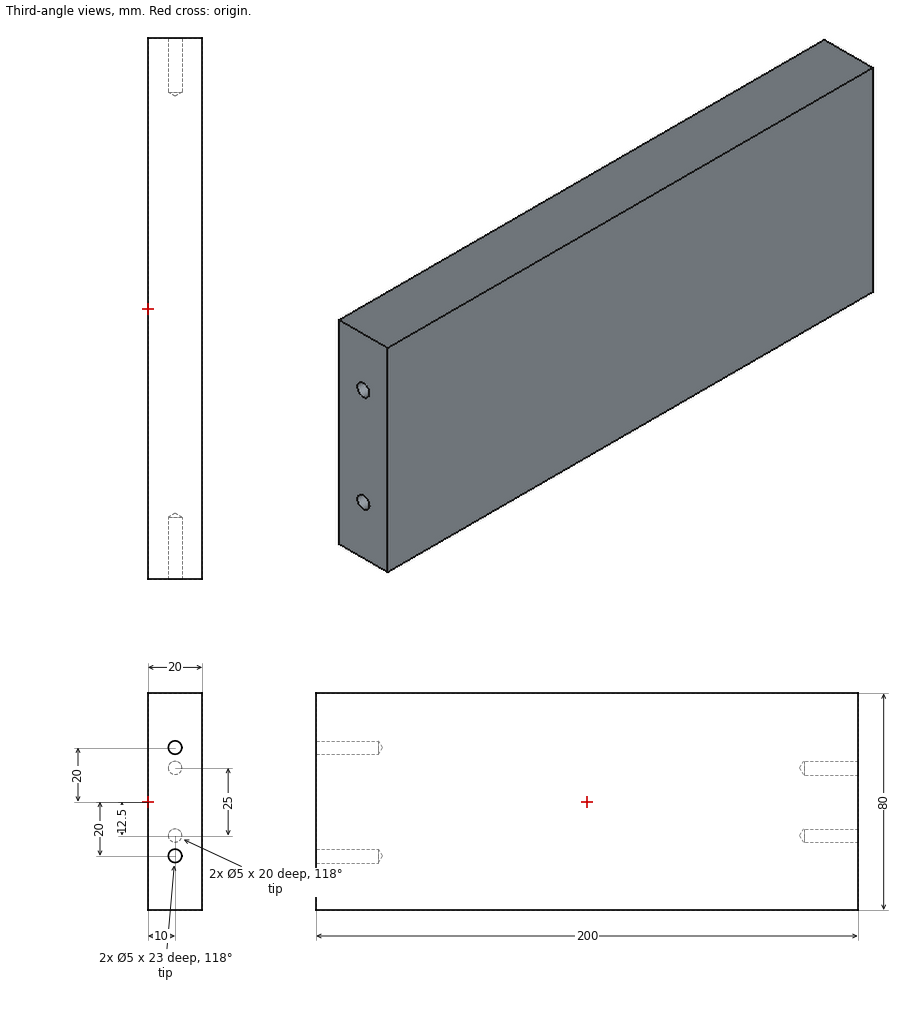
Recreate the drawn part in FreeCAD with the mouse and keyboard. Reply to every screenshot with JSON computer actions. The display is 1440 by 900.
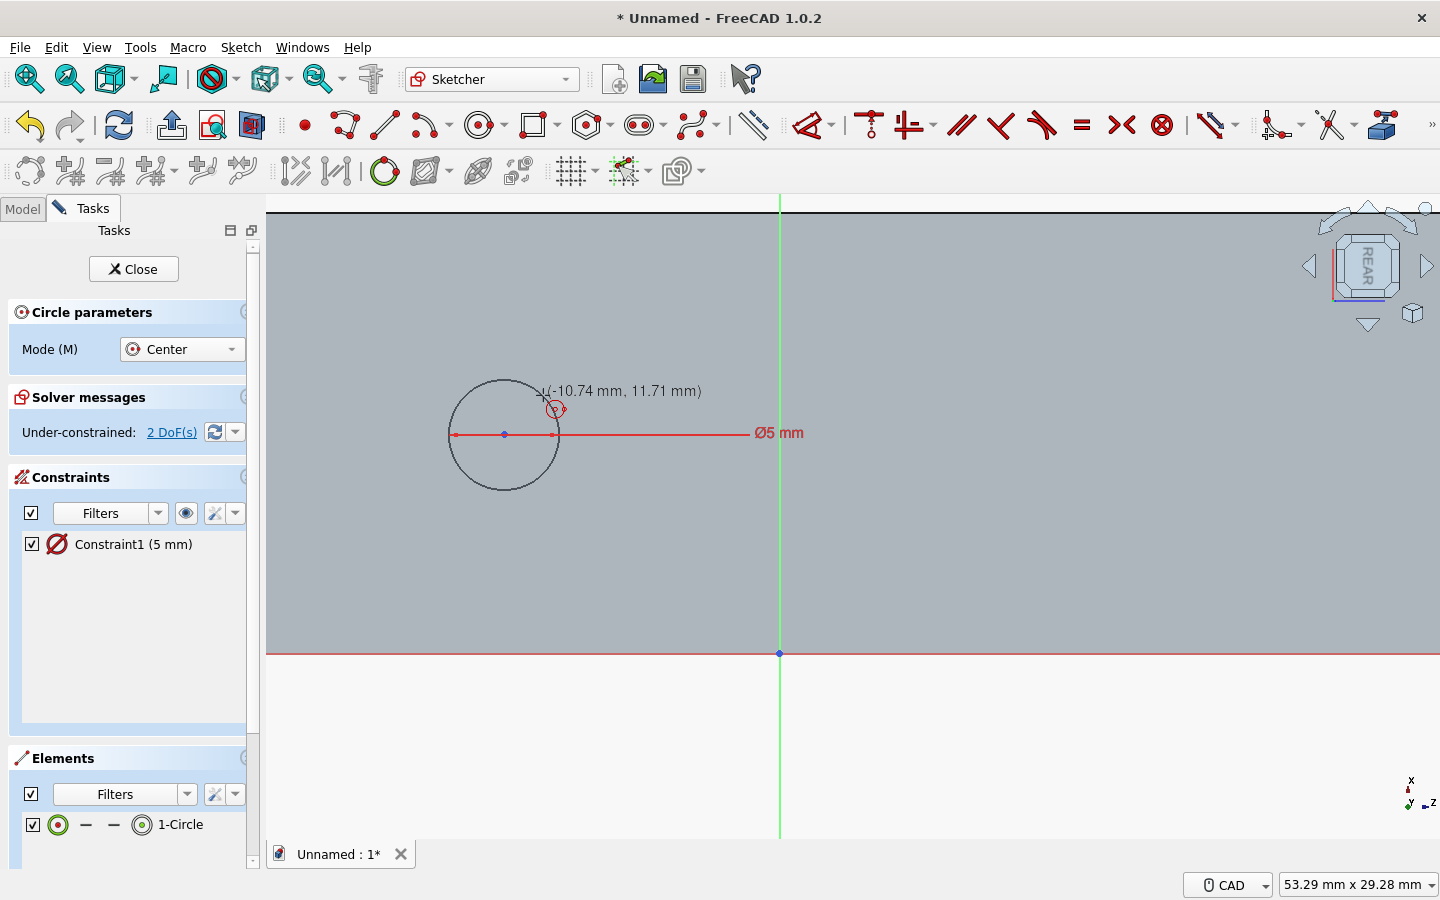
{"action": "left_click", "coordinate": [1055, 434]}
{"action": "mouse_move", "coordinate": [1094, 395]}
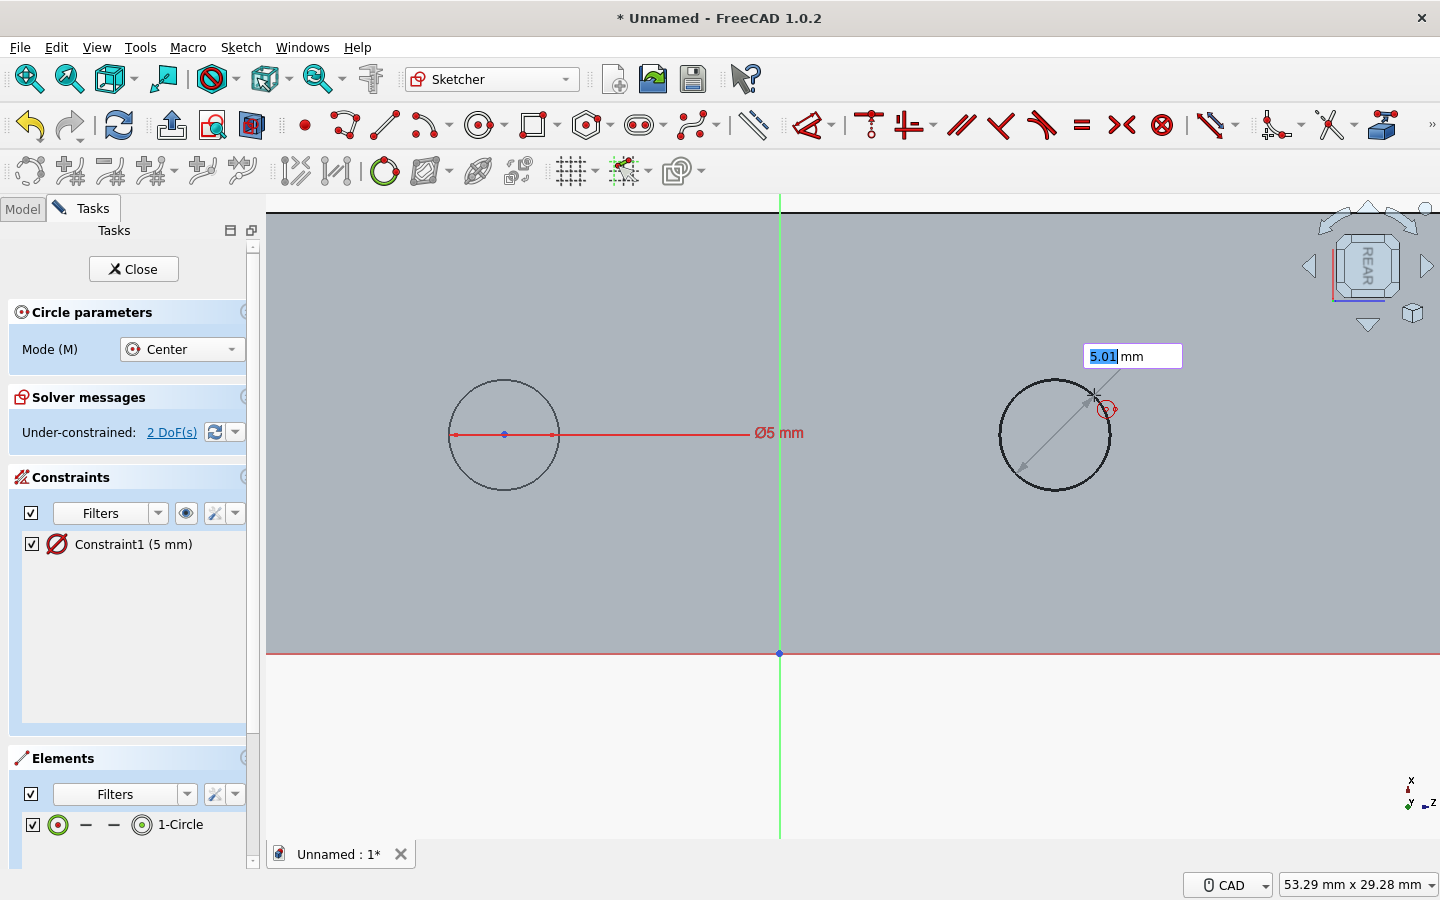
{"action": "type", "text": "5"}
{"action": "key", "text": "Return"}
{"action": "key", "text": "Escape"}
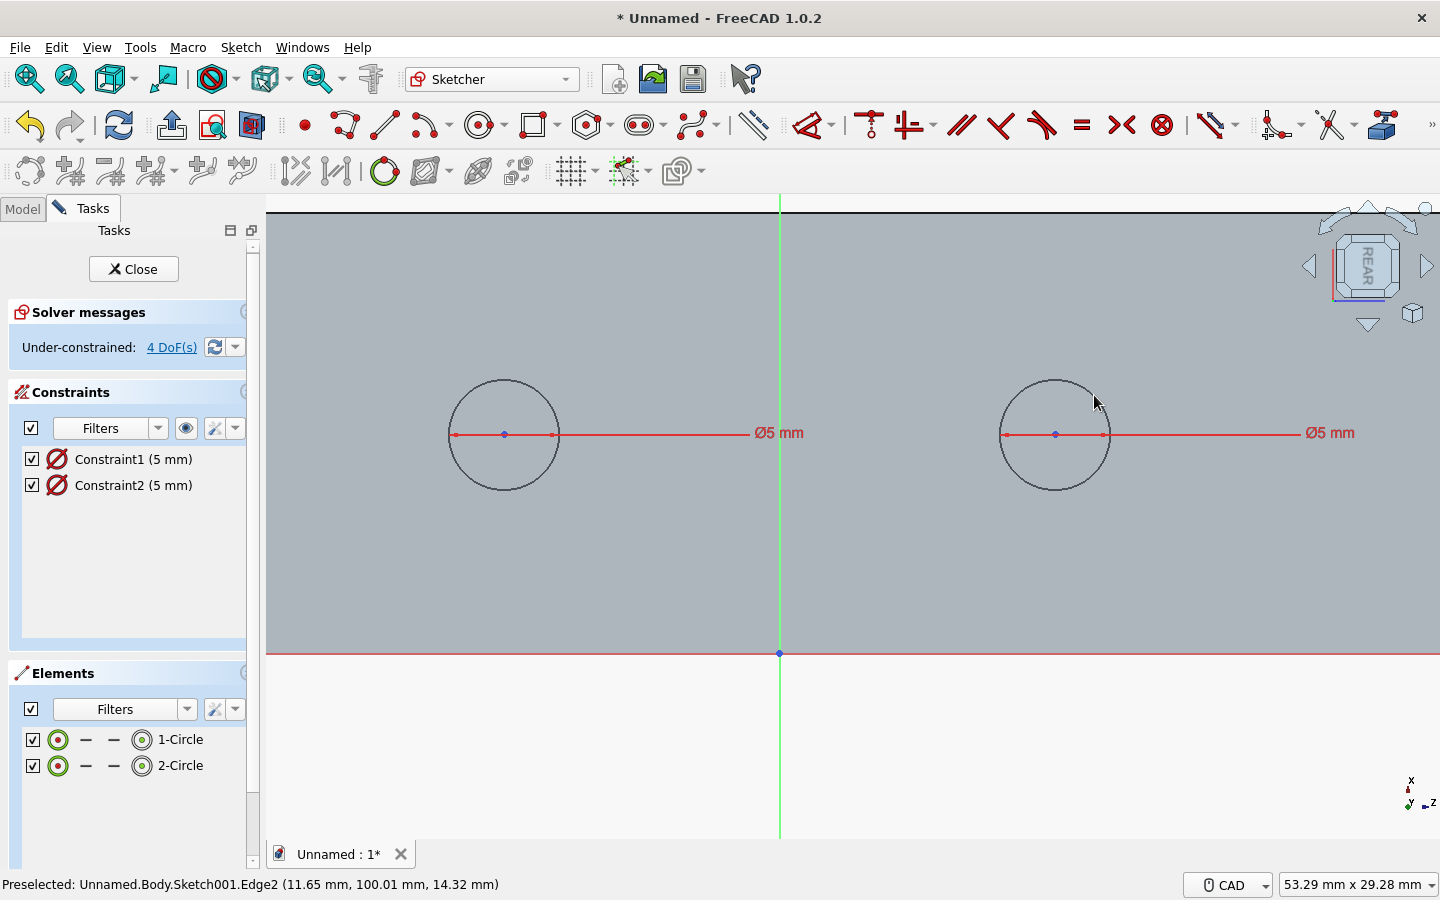
{"action": "left_click", "coordinate": [504, 435]}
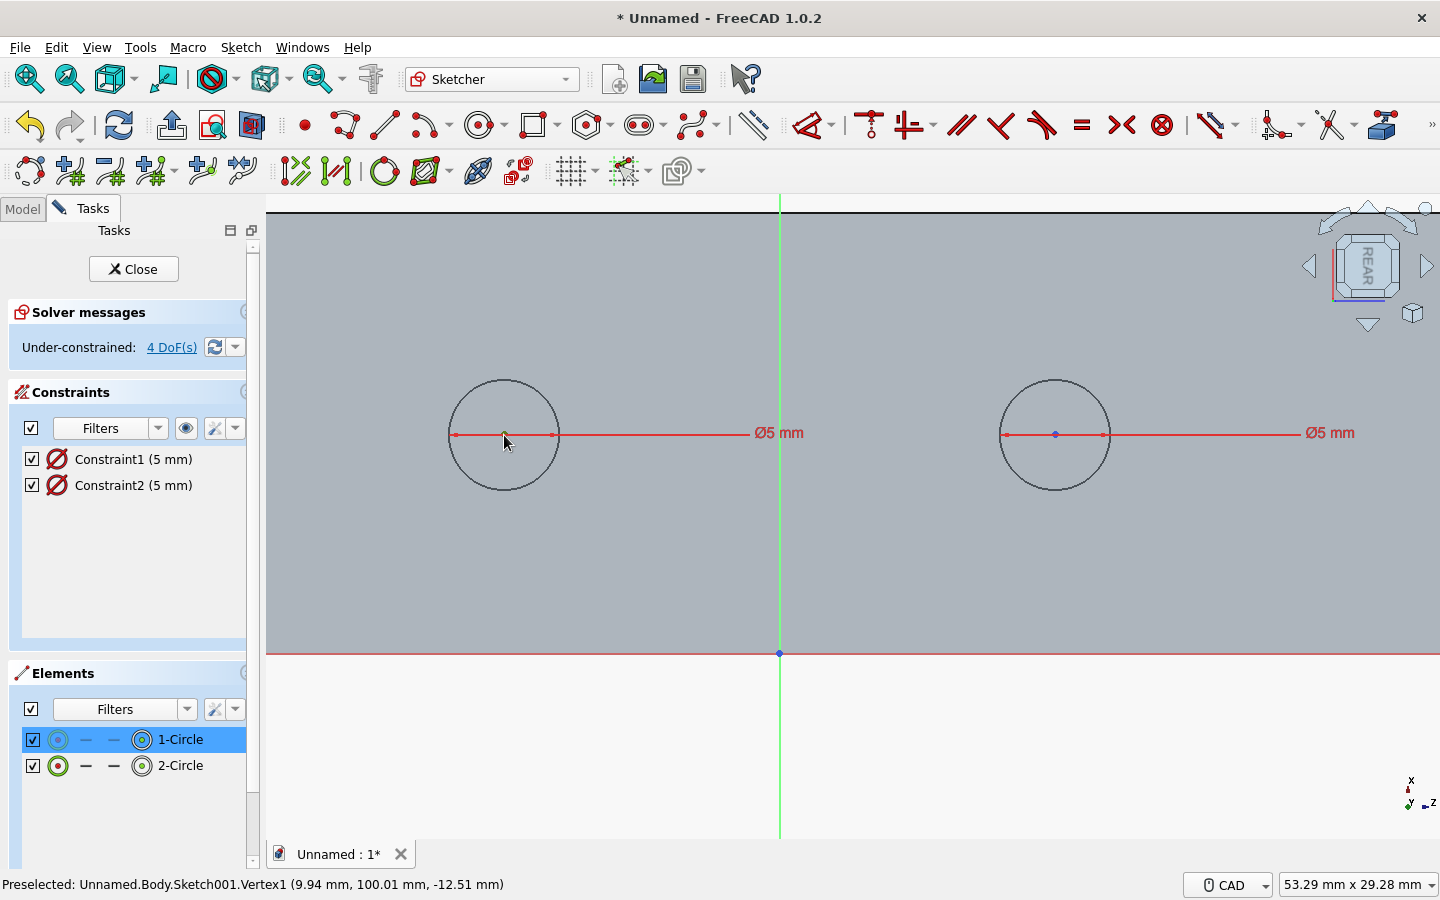
{"action": "left_click", "coordinate": [1055, 435]}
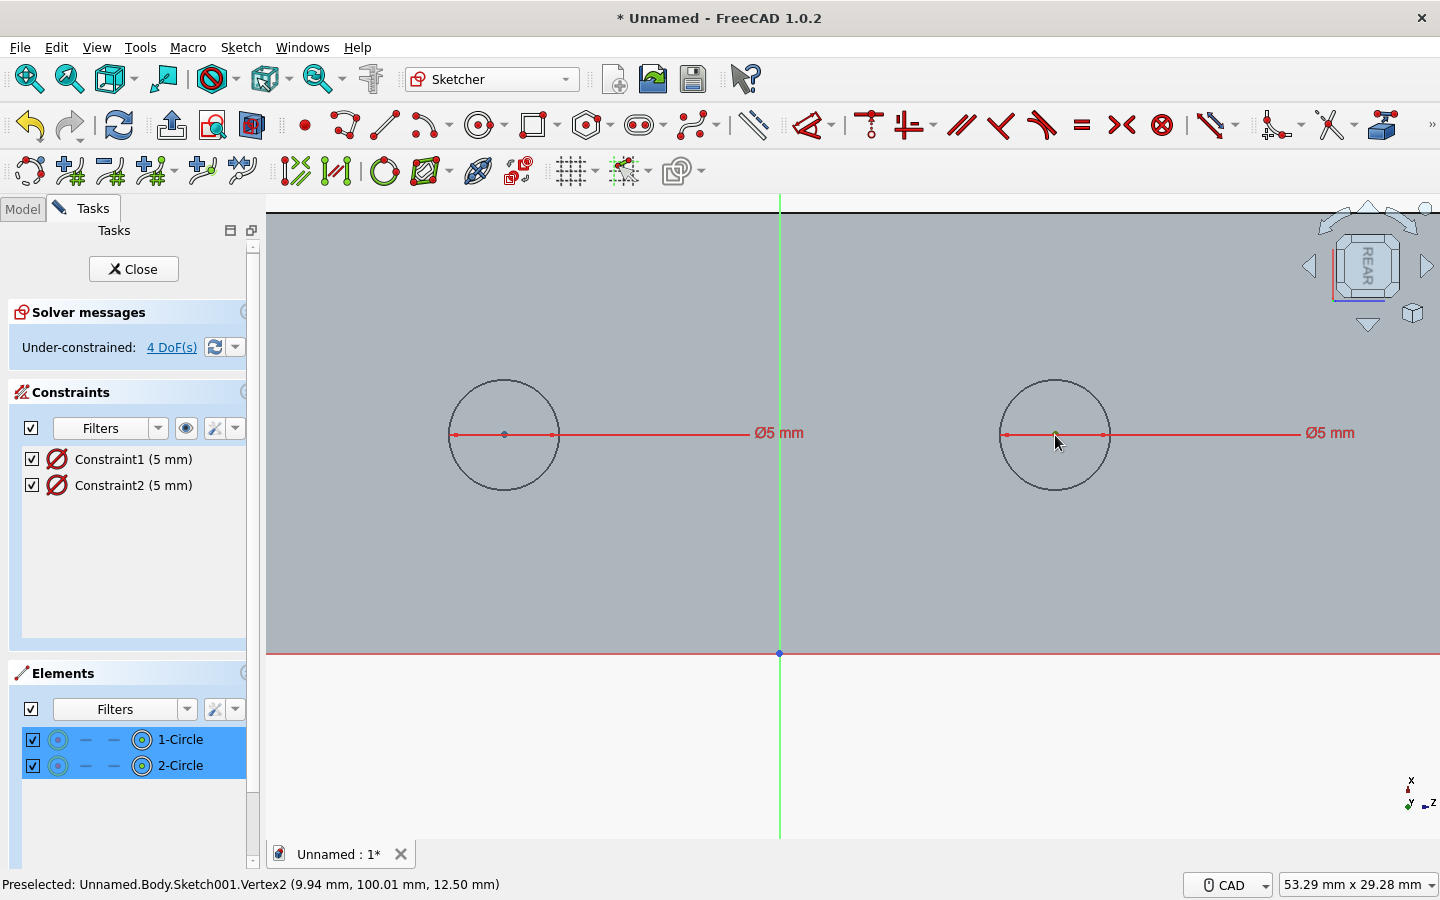
{"action": "key", "text": "h"}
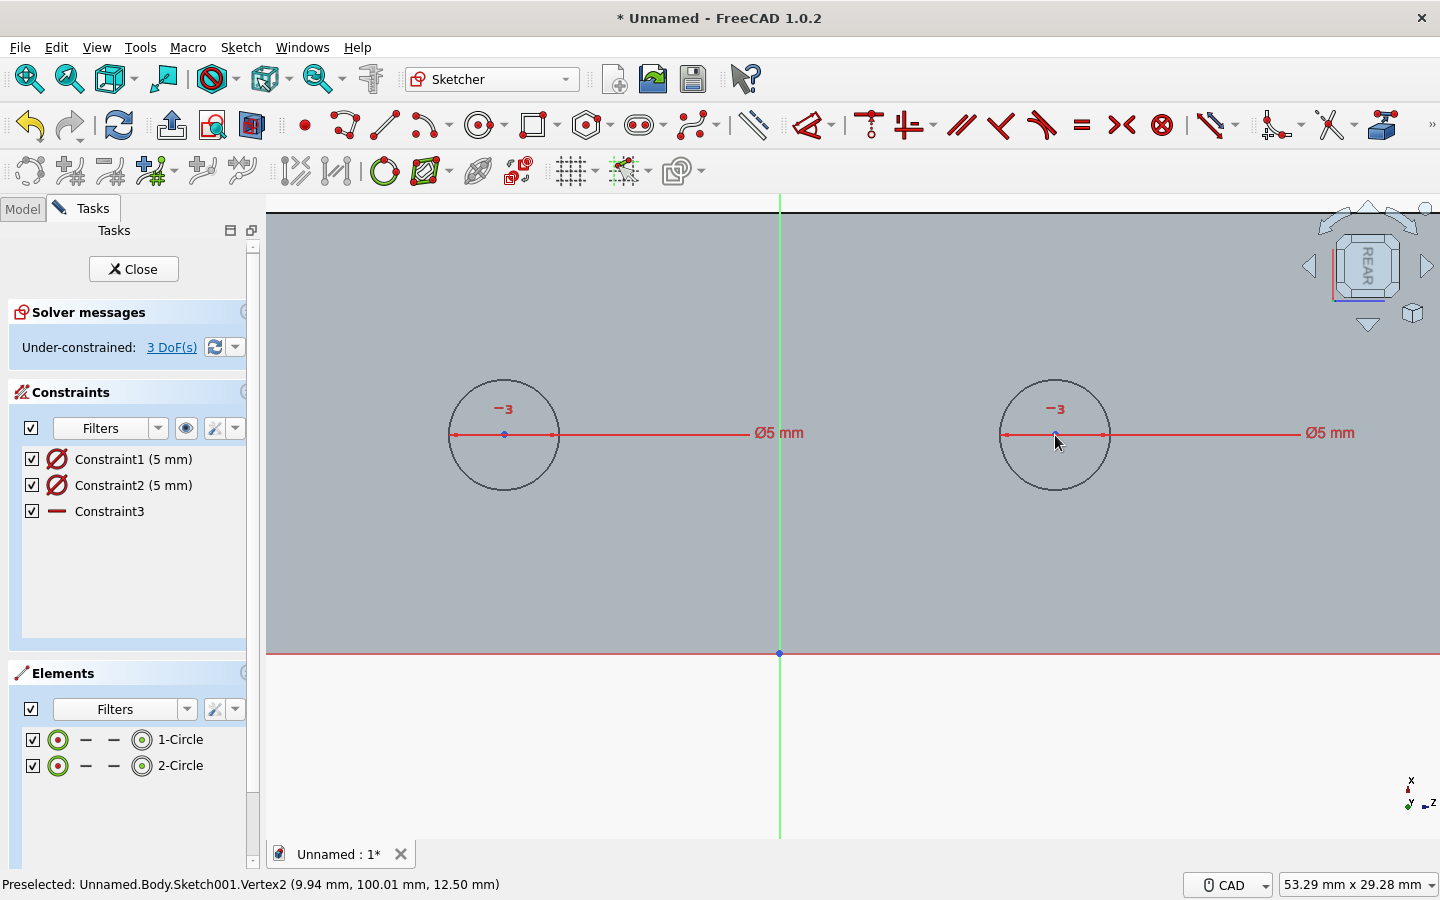
{"action": "key", "text": "d"}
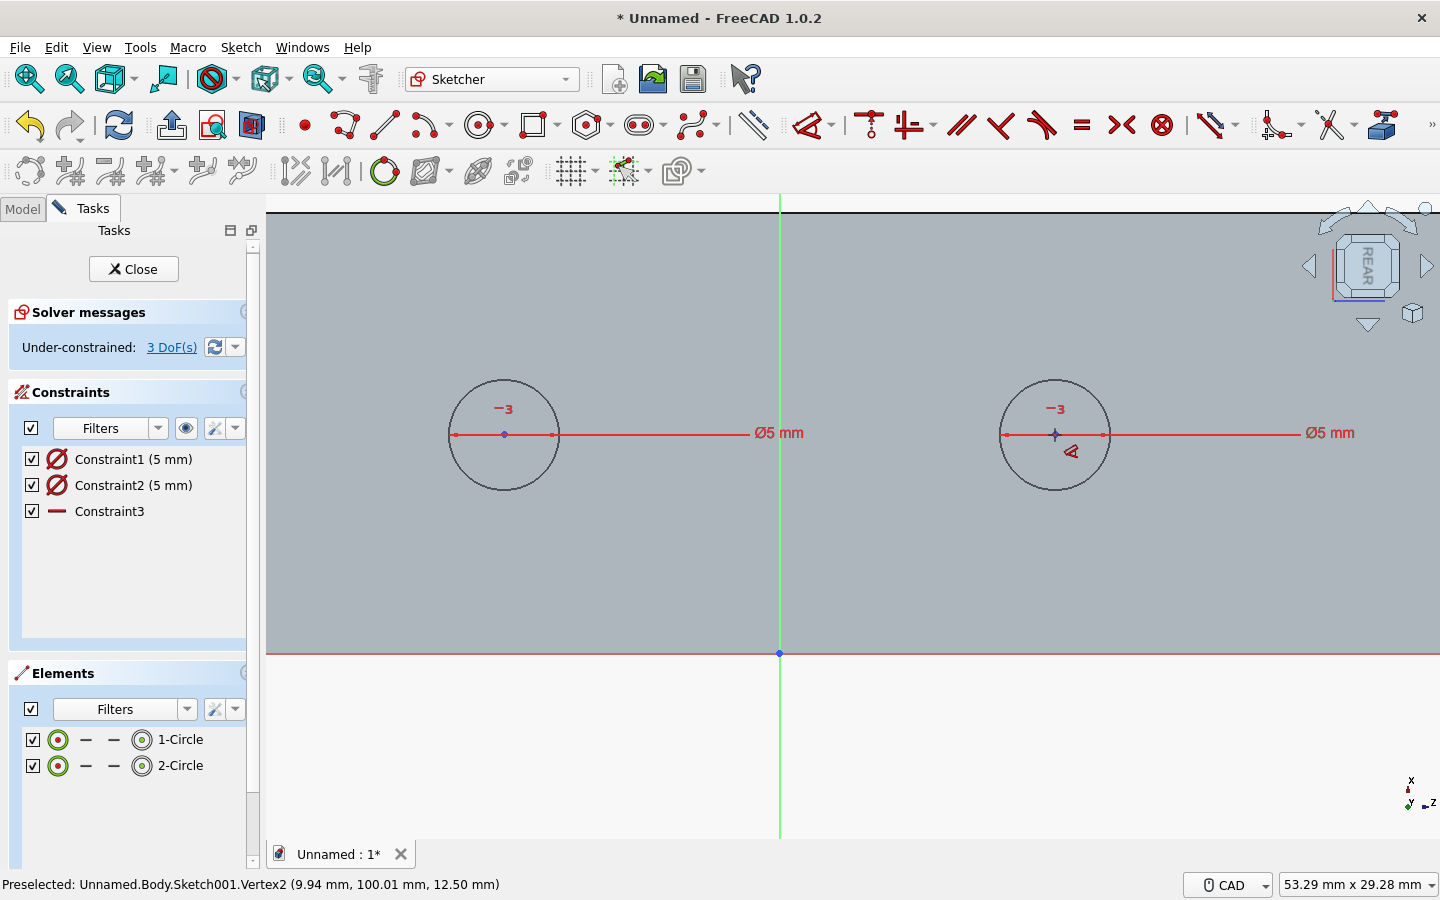
{"action": "left_click", "coordinate": [504, 435]}
{"action": "left_click", "coordinate": [470, 544]}